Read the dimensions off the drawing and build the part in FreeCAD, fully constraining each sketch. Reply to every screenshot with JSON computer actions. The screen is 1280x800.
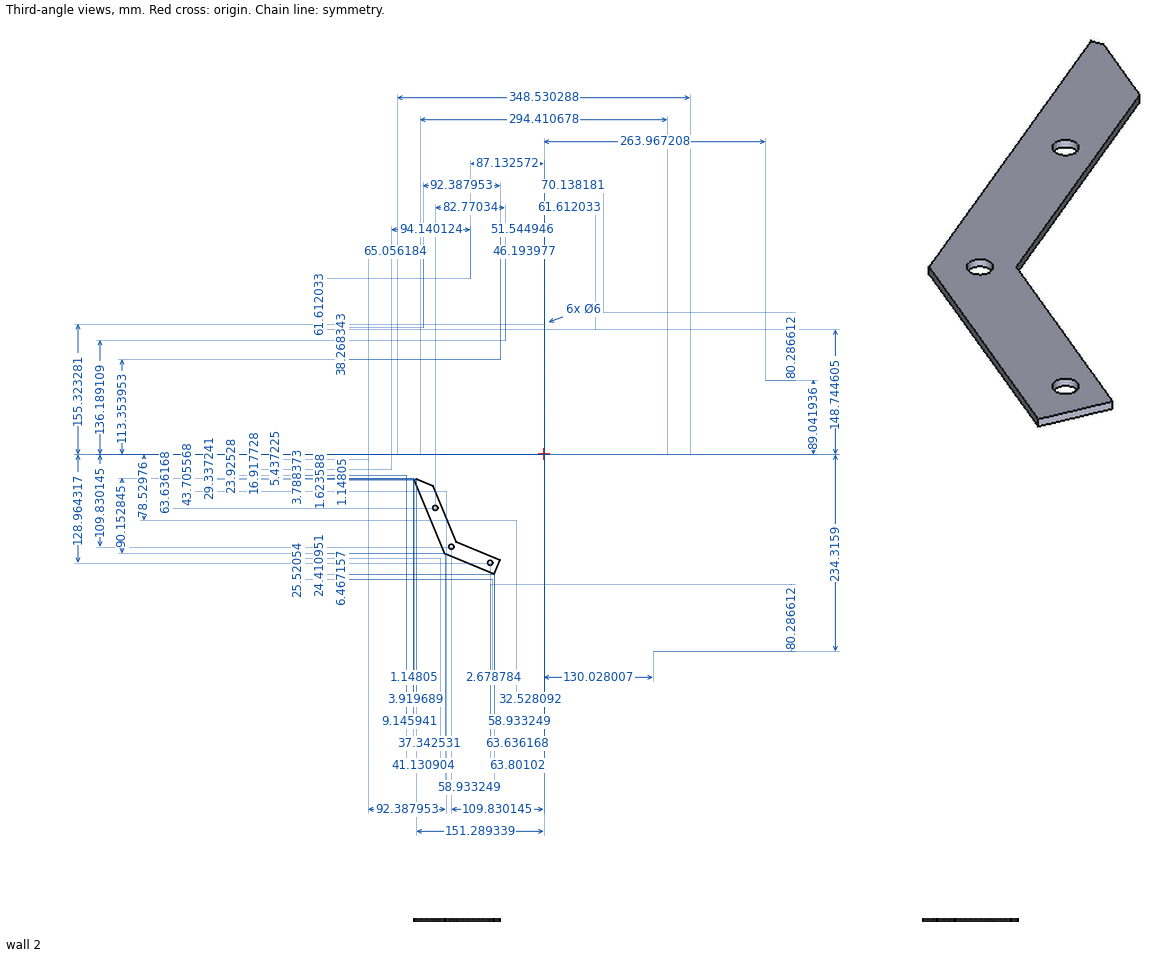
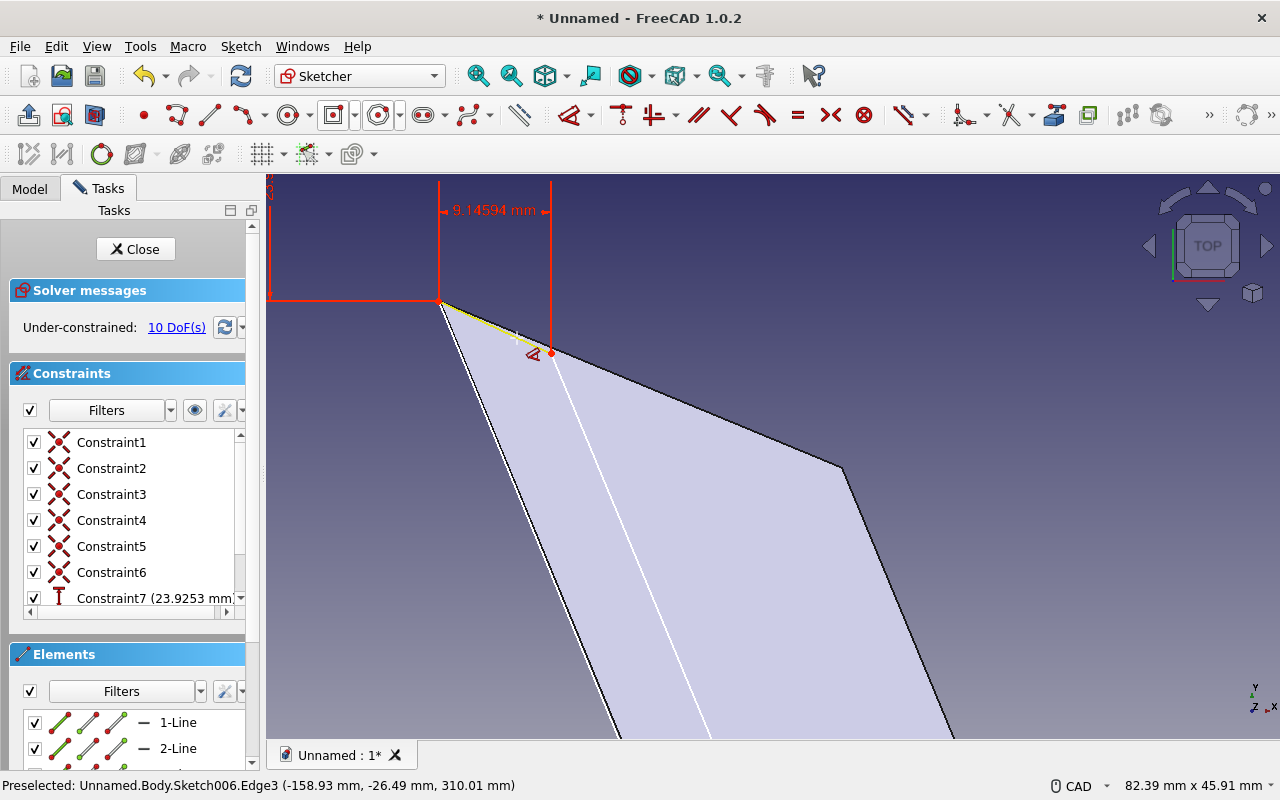
{"action": "left_click", "coordinate": [517, 338]}
{"action": "left_click", "coordinate": [405, 328]}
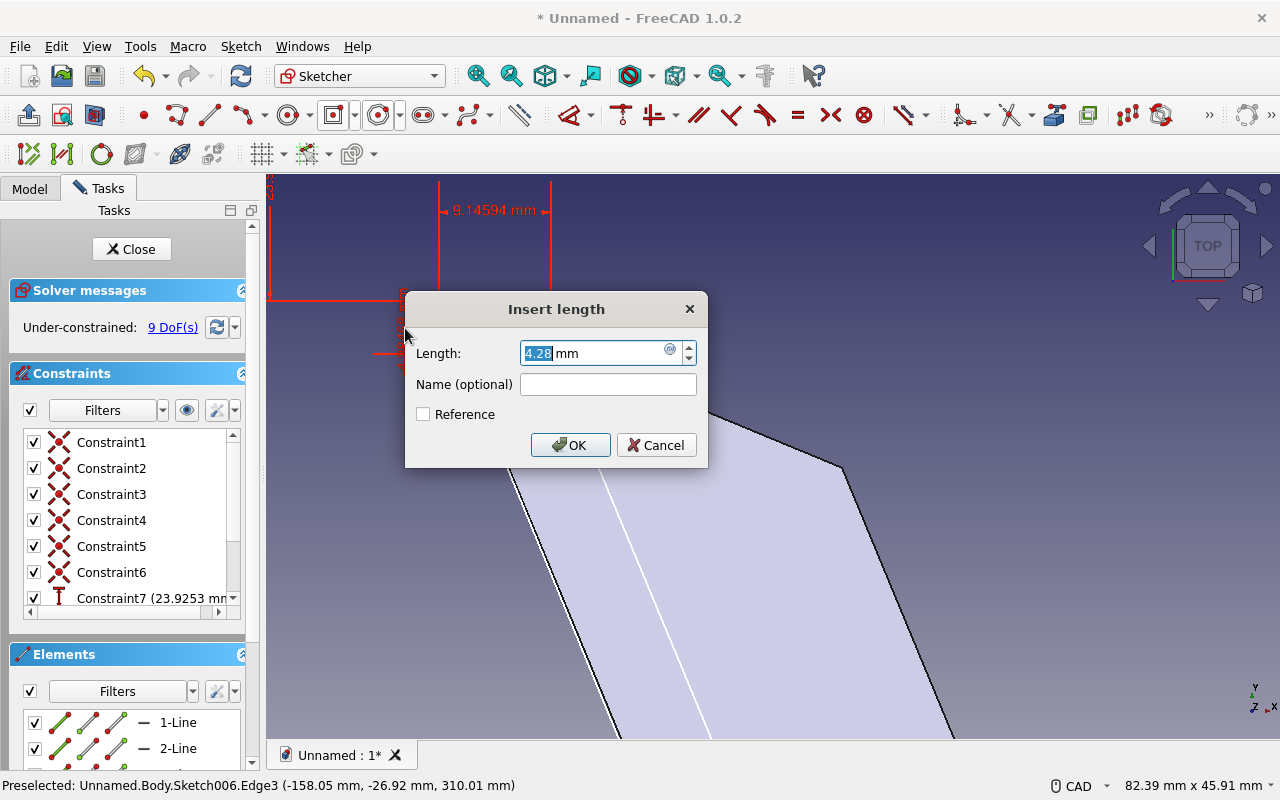
{"action": "type", "text": "3.788373"}
{"action": "key", "text": "Return"}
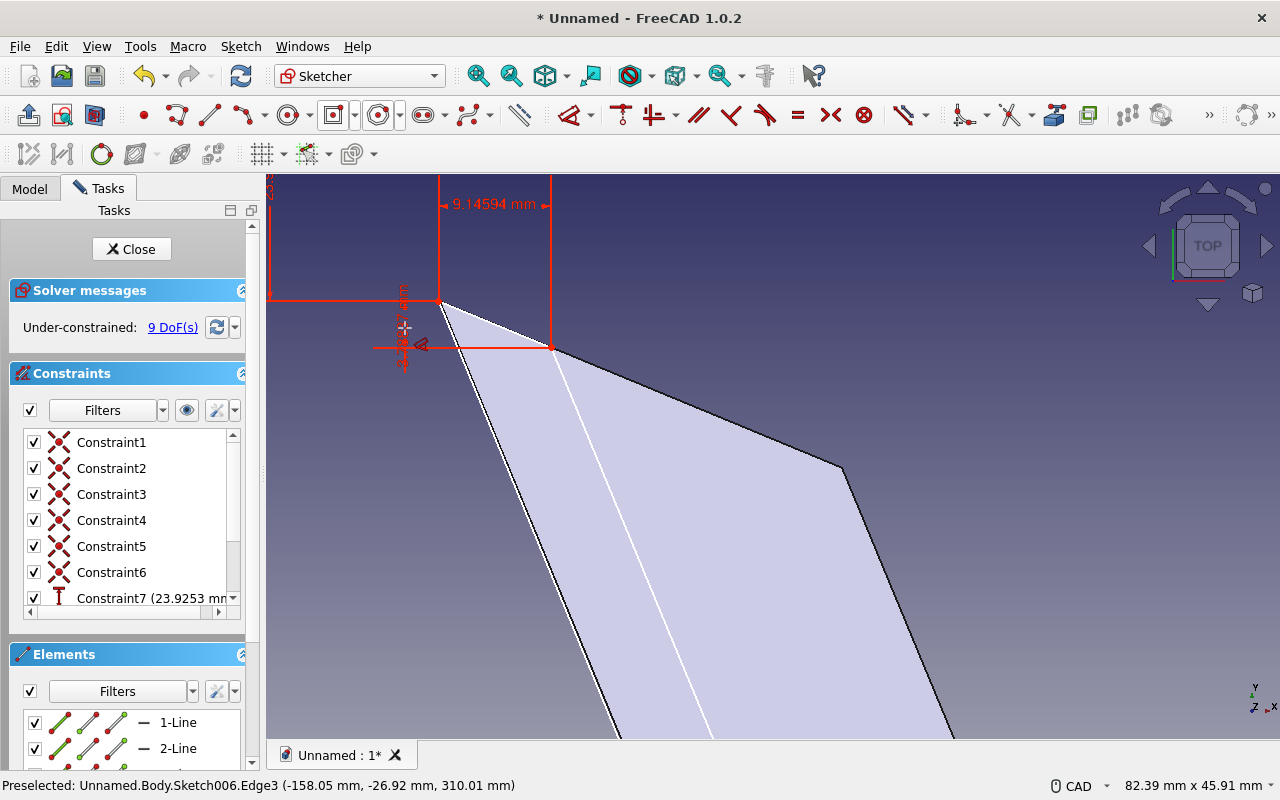
{"action": "scroll", "coordinate": [516, 339], "scroll_direction": "down", "scroll_amount": 8}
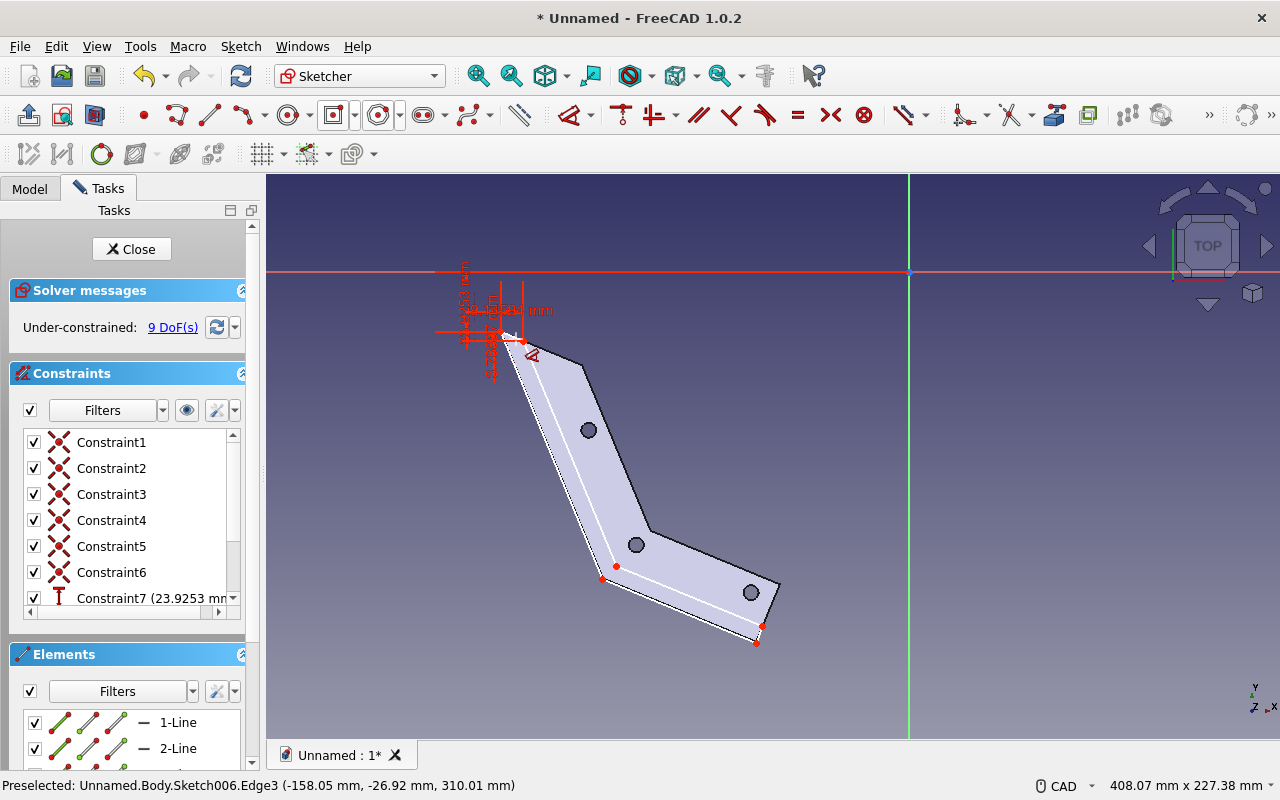
{"action": "left_click", "coordinate": [649, 598]}
{"action": "left_click", "coordinate": [569, 611]}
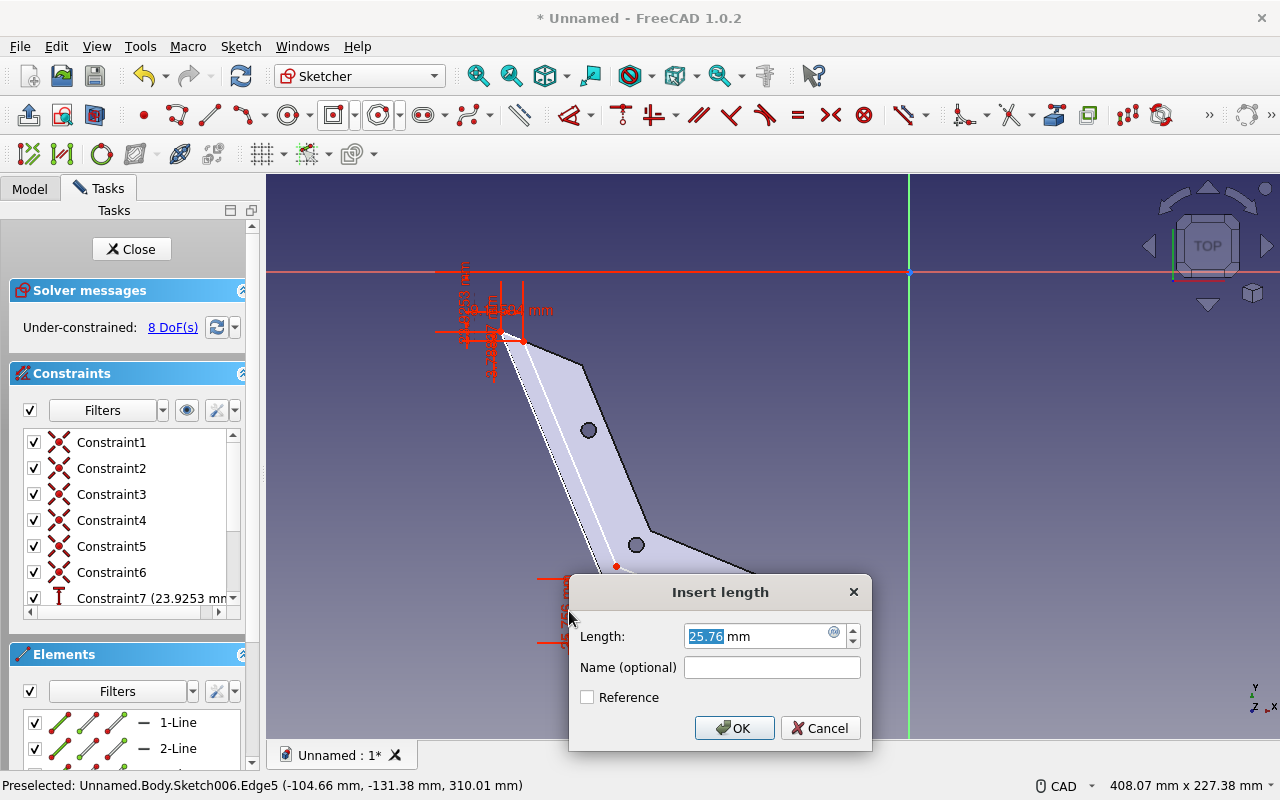
{"action": "type", "text": "25.52054"}
{"action": "key", "text": "Return"}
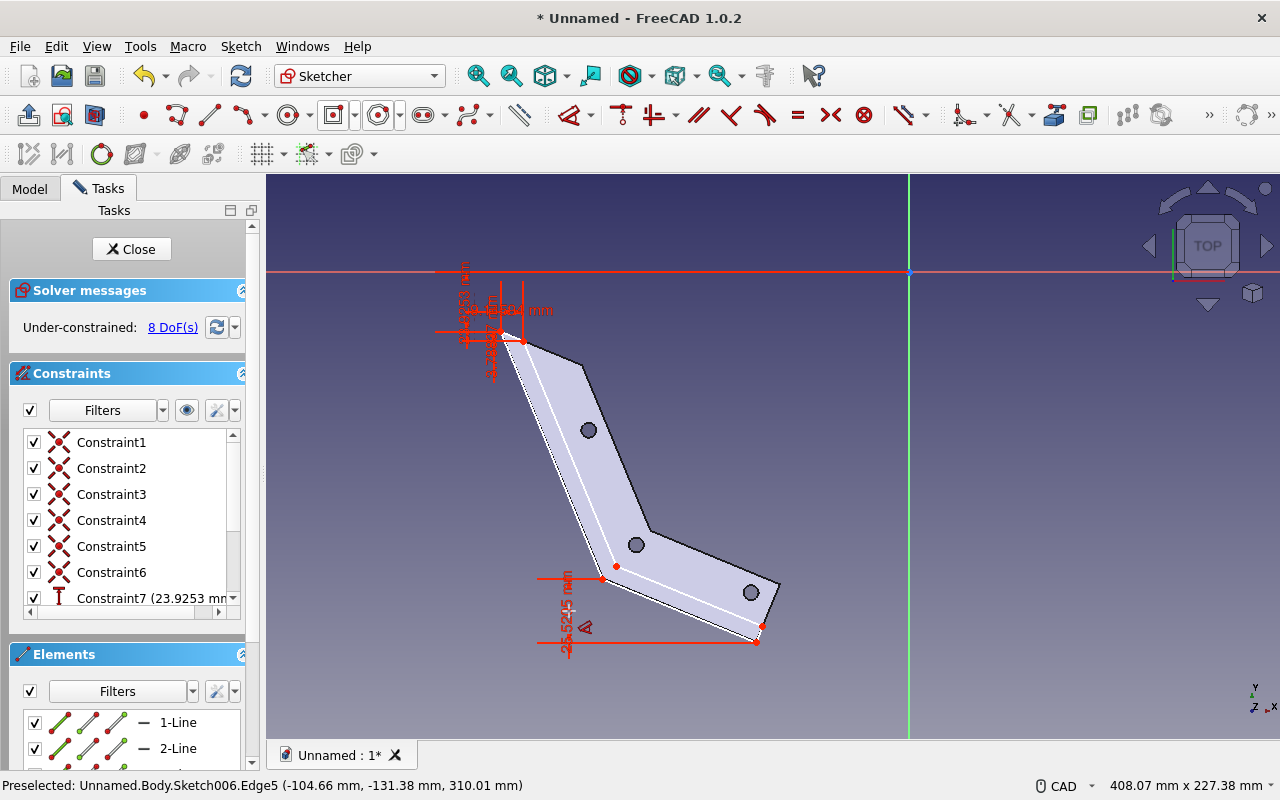
{"action": "scroll", "coordinate": [760, 635], "scroll_direction": "up", "scroll_amount": 9}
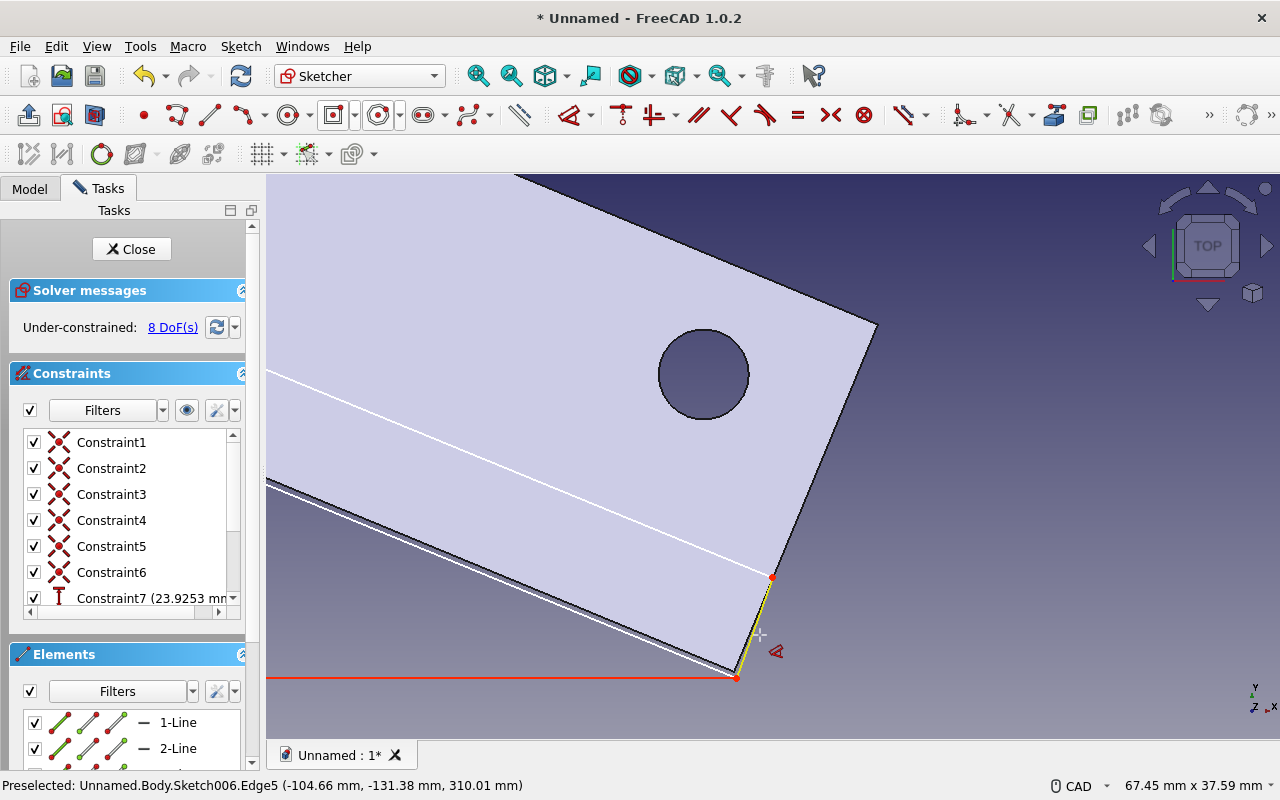
{"action": "left_click", "coordinate": [755, 628]}
{"action": "left_click", "coordinate": [755, 544]}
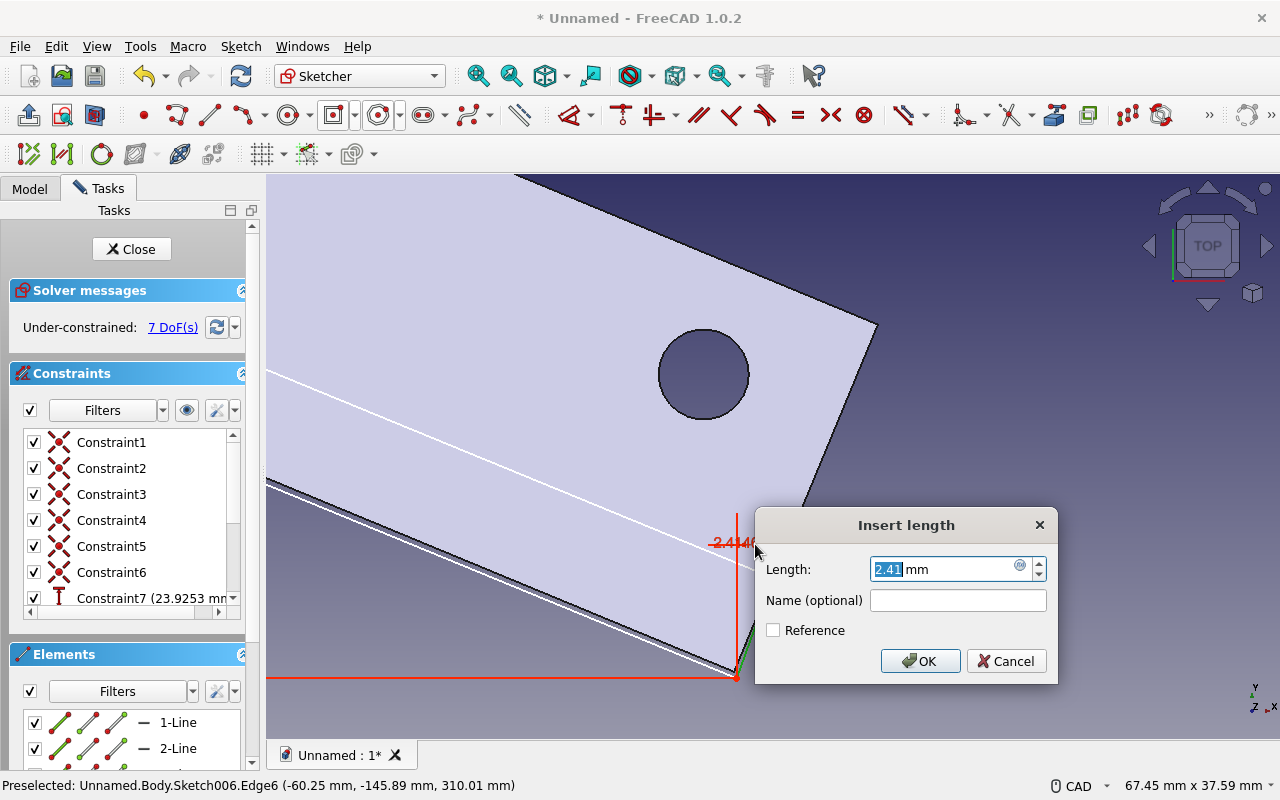
{"action": "type", "text": "2.678784"}
{"action": "key", "text": "Return"}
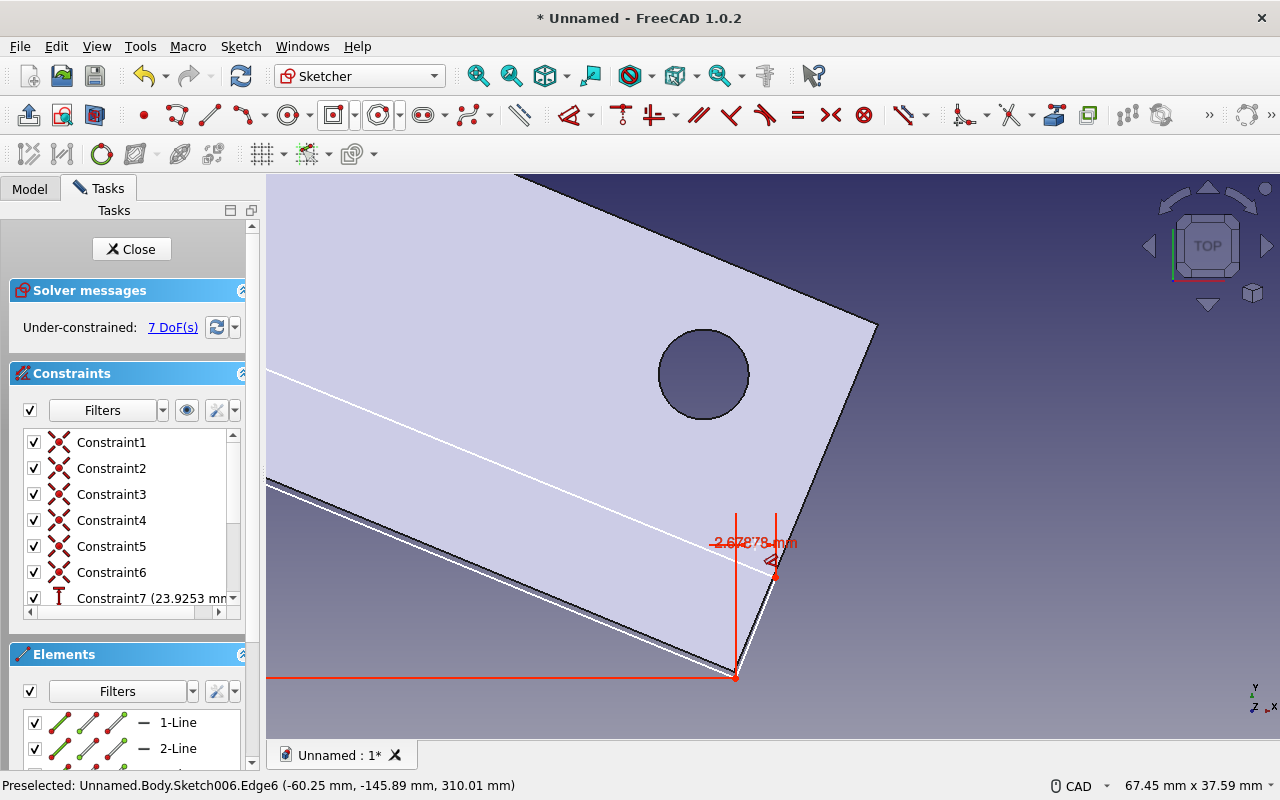
{"action": "left_click", "coordinate": [748, 648]}
{"action": "left_click", "coordinate": [810, 628]}